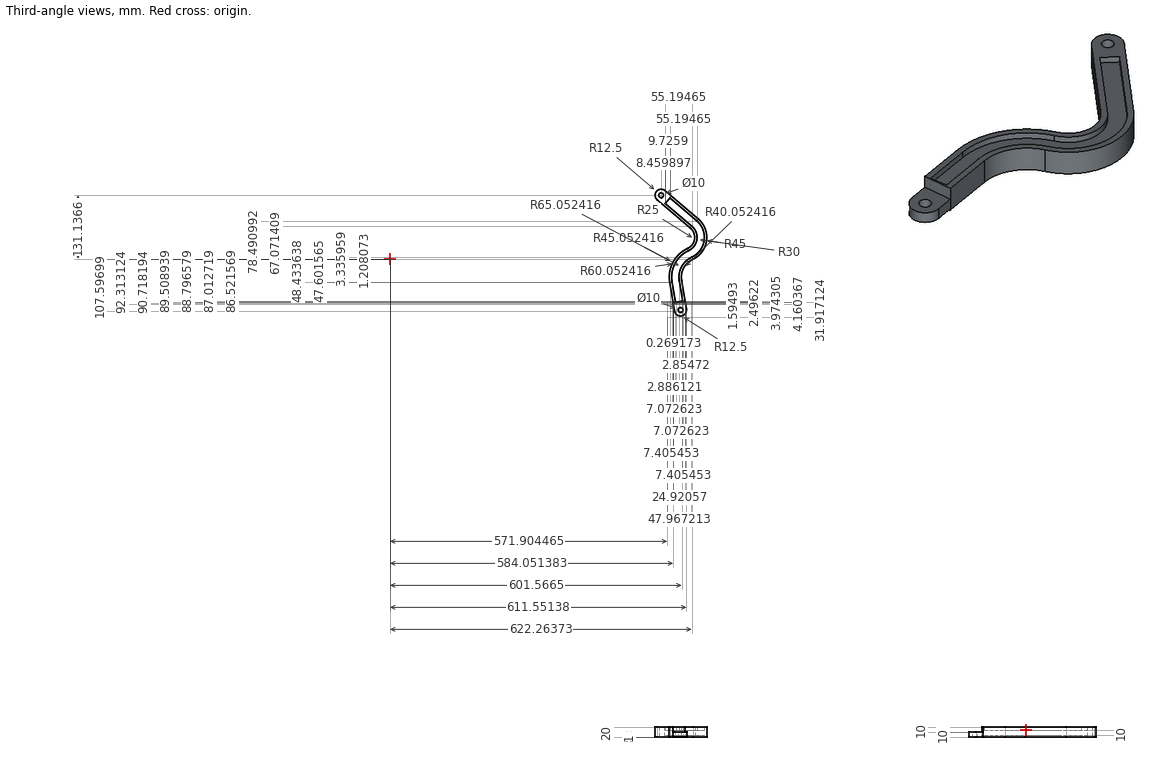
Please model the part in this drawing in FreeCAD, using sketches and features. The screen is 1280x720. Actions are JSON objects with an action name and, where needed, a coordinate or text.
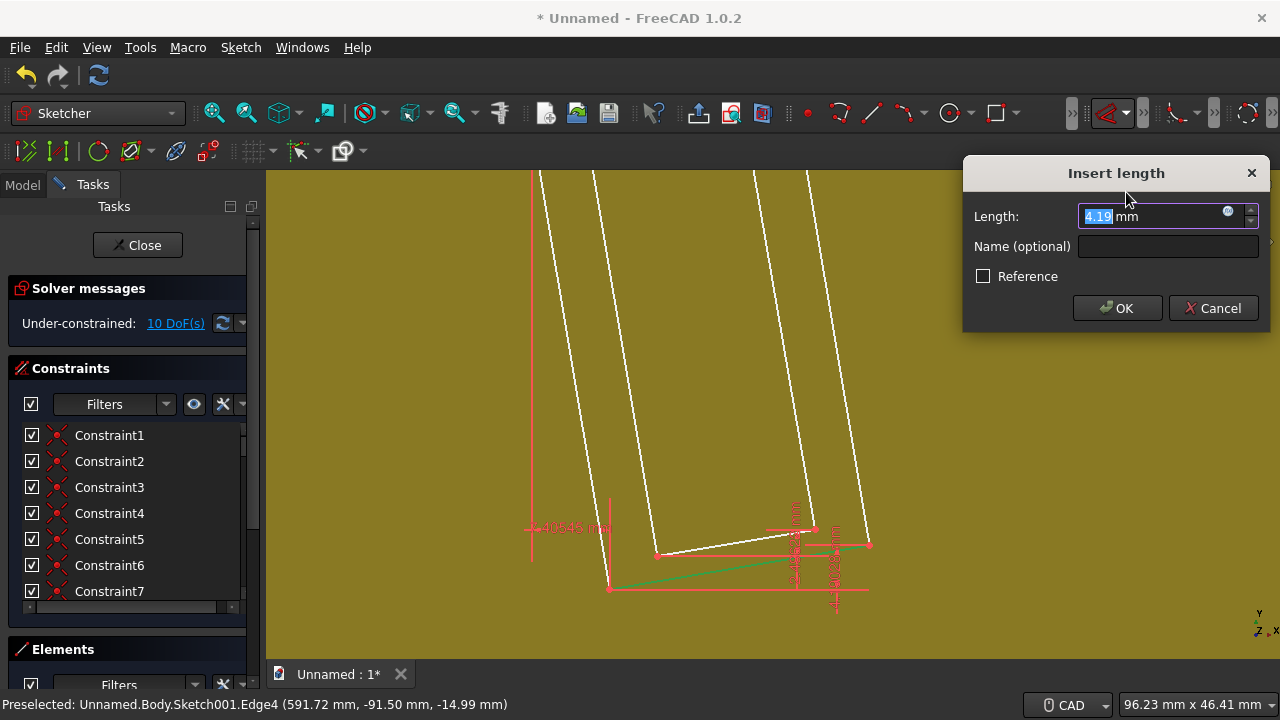
{"action": "type", "text": "4.160367"}
{"action": "key", "text": "Return"}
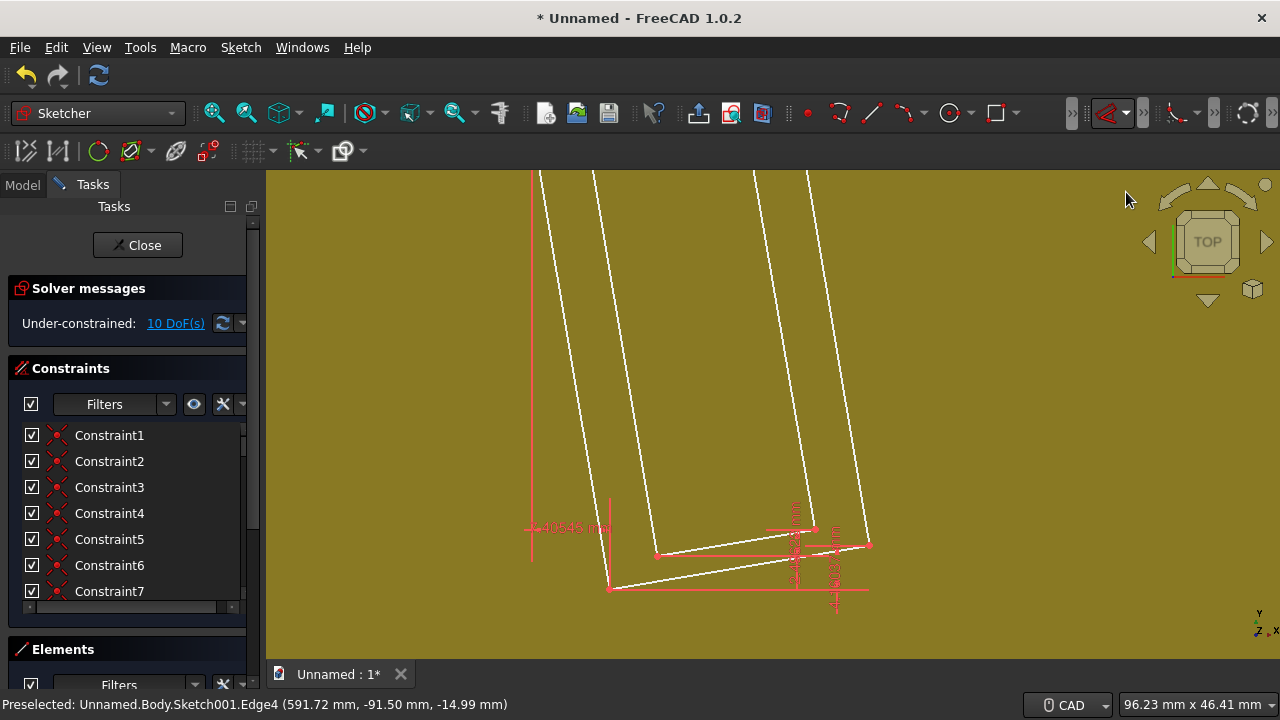
{"action": "left_click", "coordinate": [846, 406]}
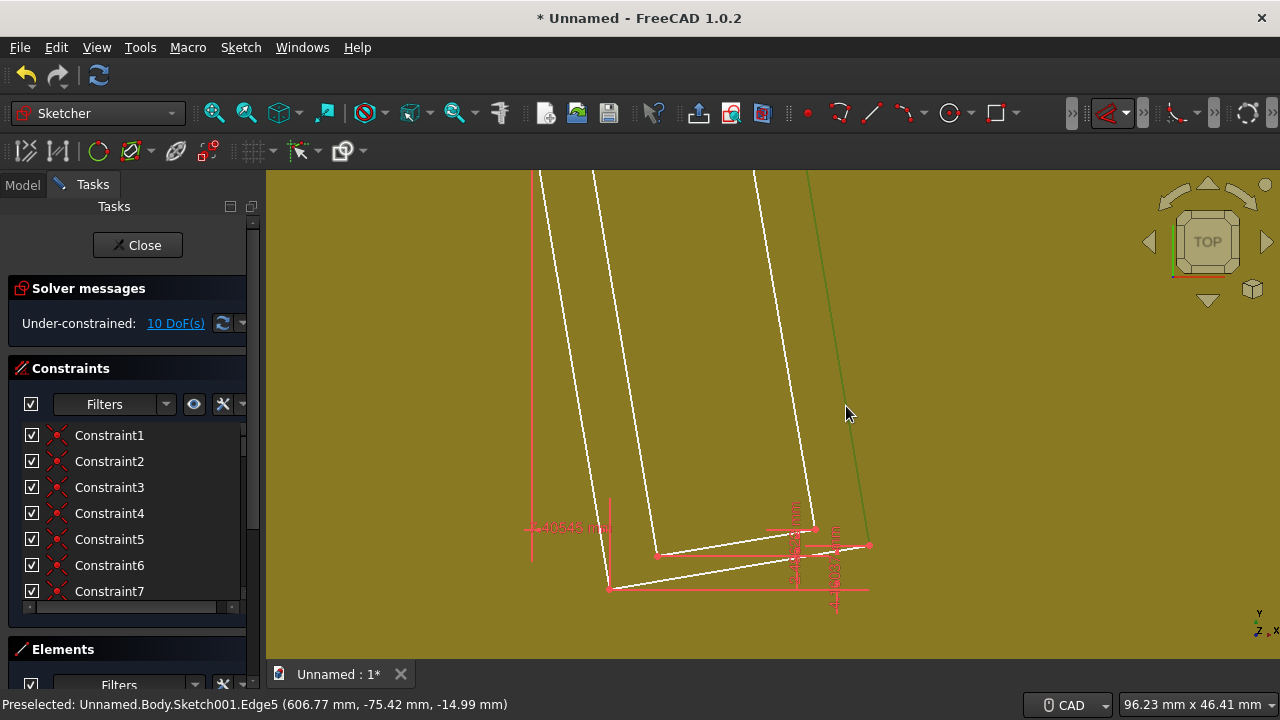
{"action": "left_click", "coordinate": [1128, 114]}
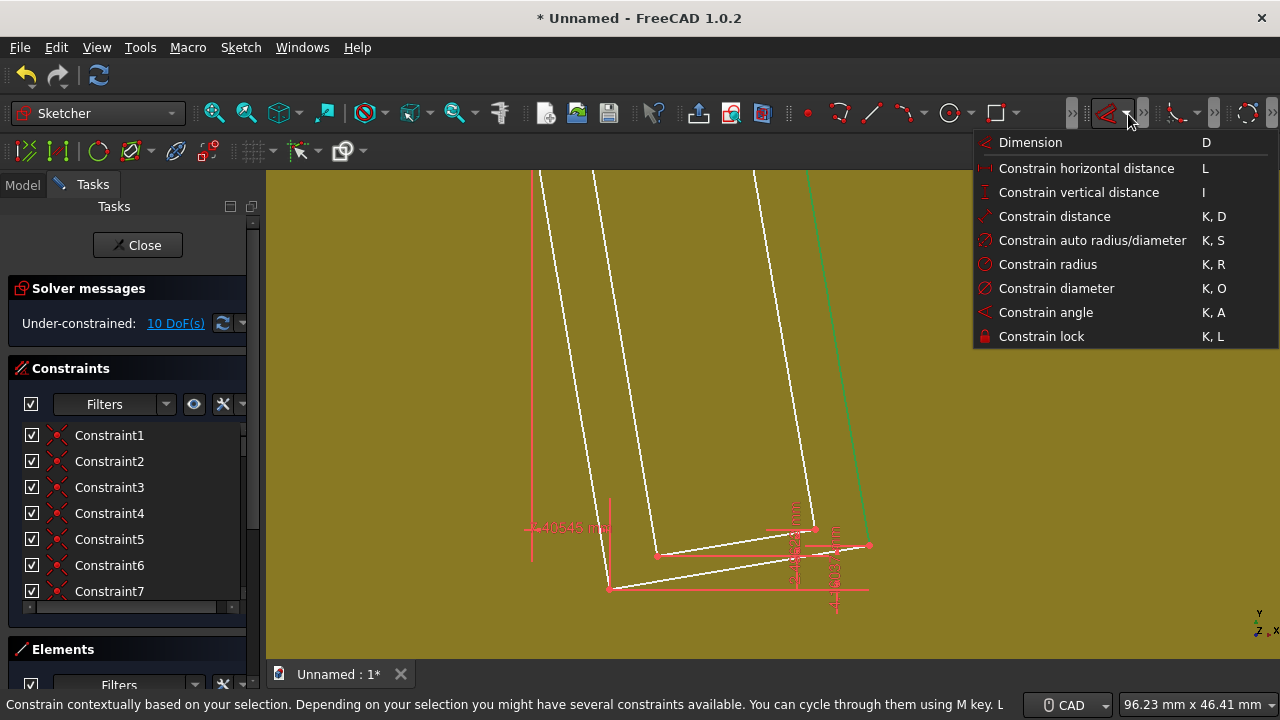
{"action": "left_click", "coordinate": [1126, 168]}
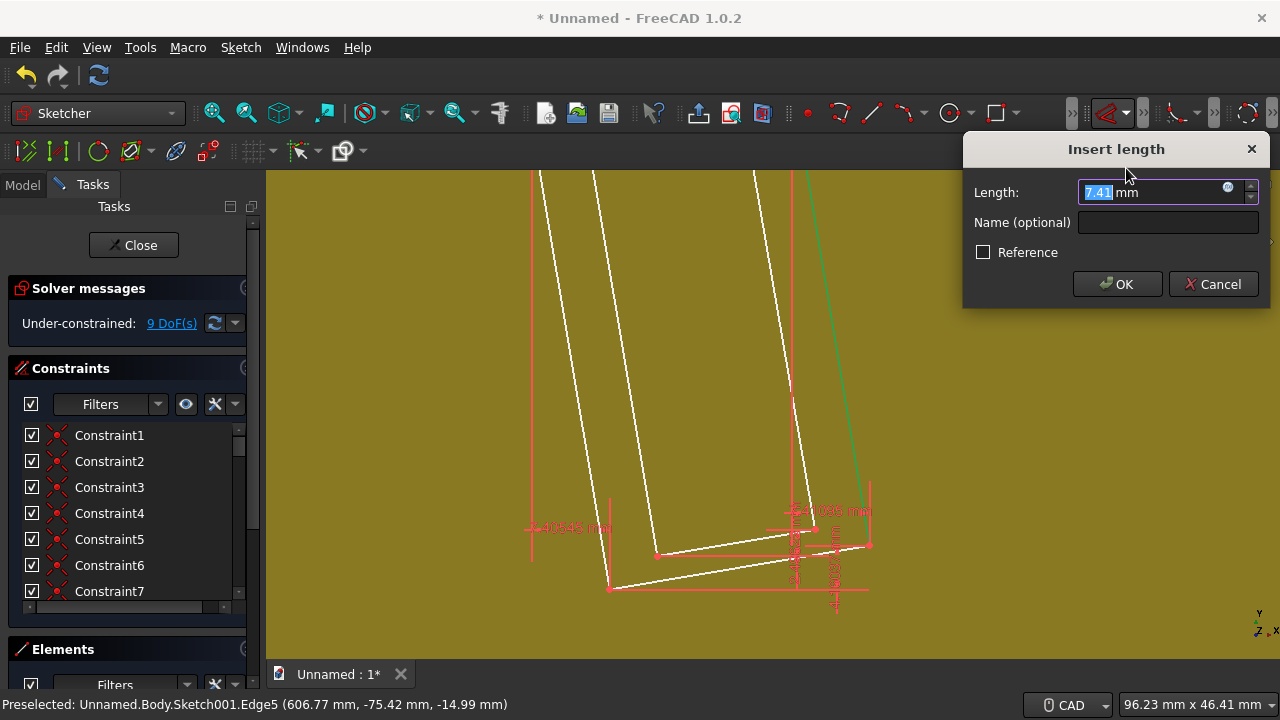
{"action": "type", "text": "7.405453"}
{"action": "key", "text": "Return"}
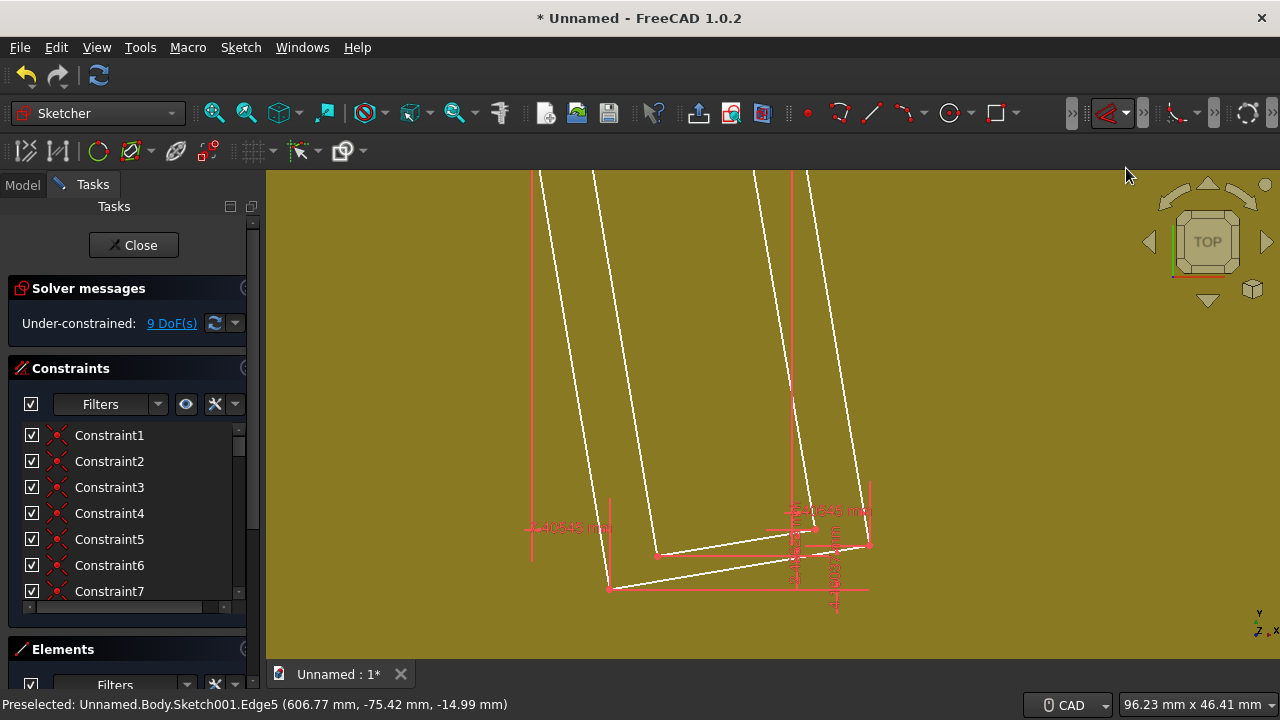
{"action": "left_click", "coordinate": [763, 223]}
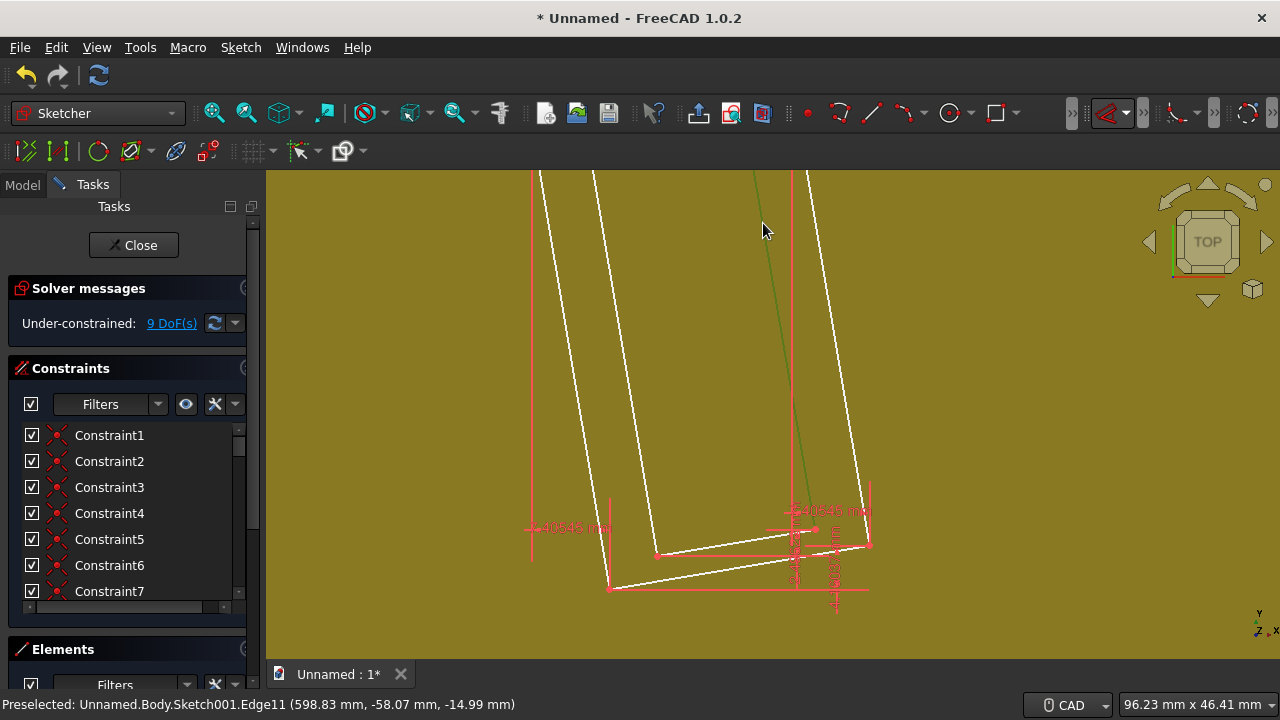
{"action": "left_click", "coordinate": [1128, 114]}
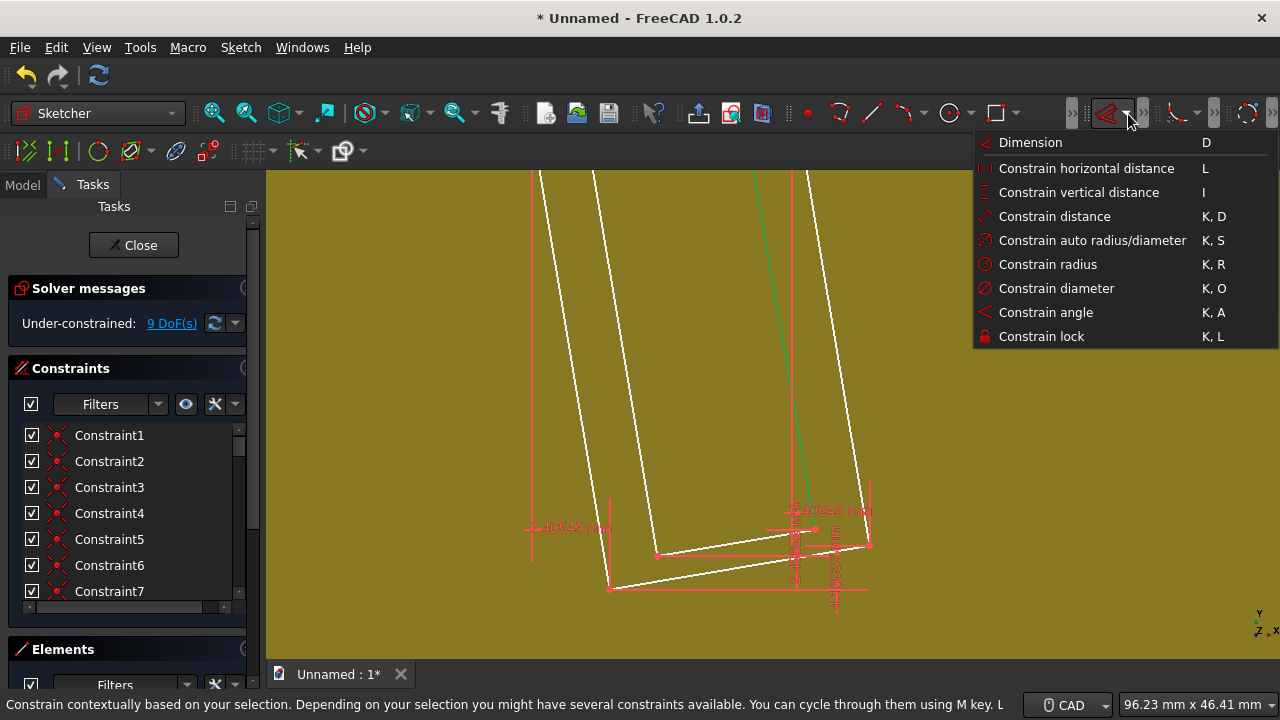
{"action": "left_click", "coordinate": [1126, 168]}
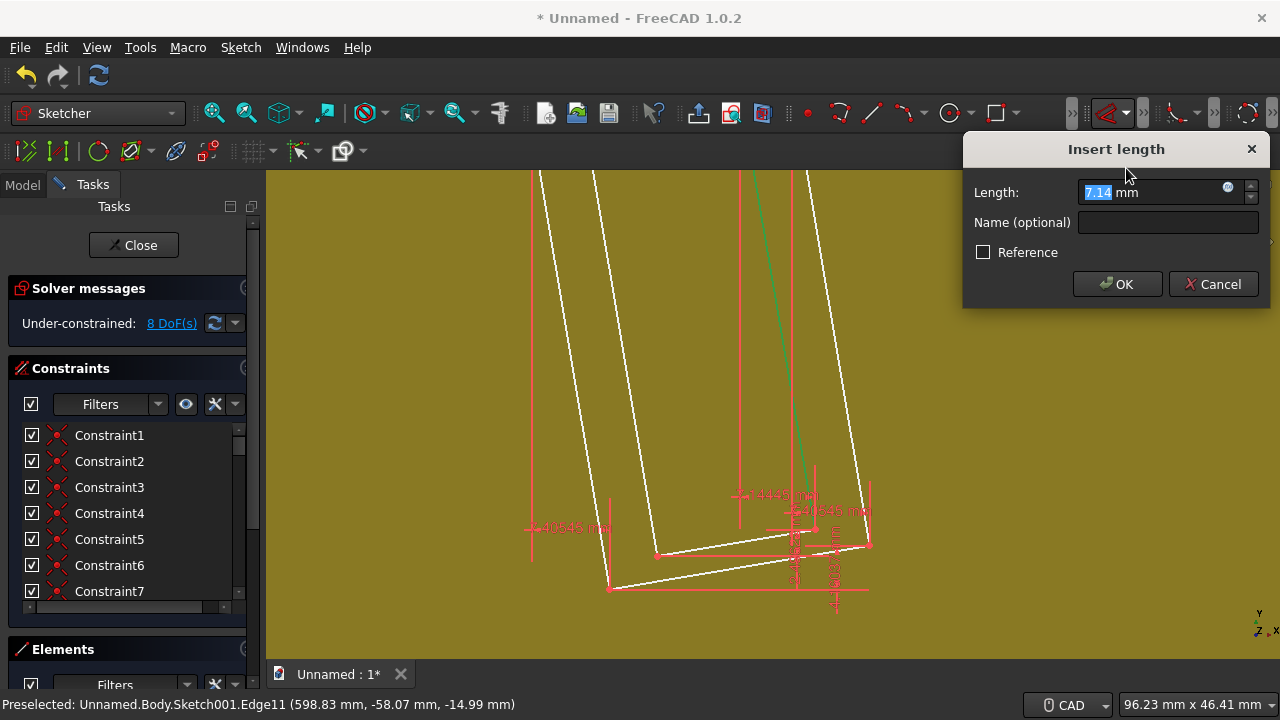
{"action": "type", "text": "7.072623"}
{"action": "key", "text": "Return"}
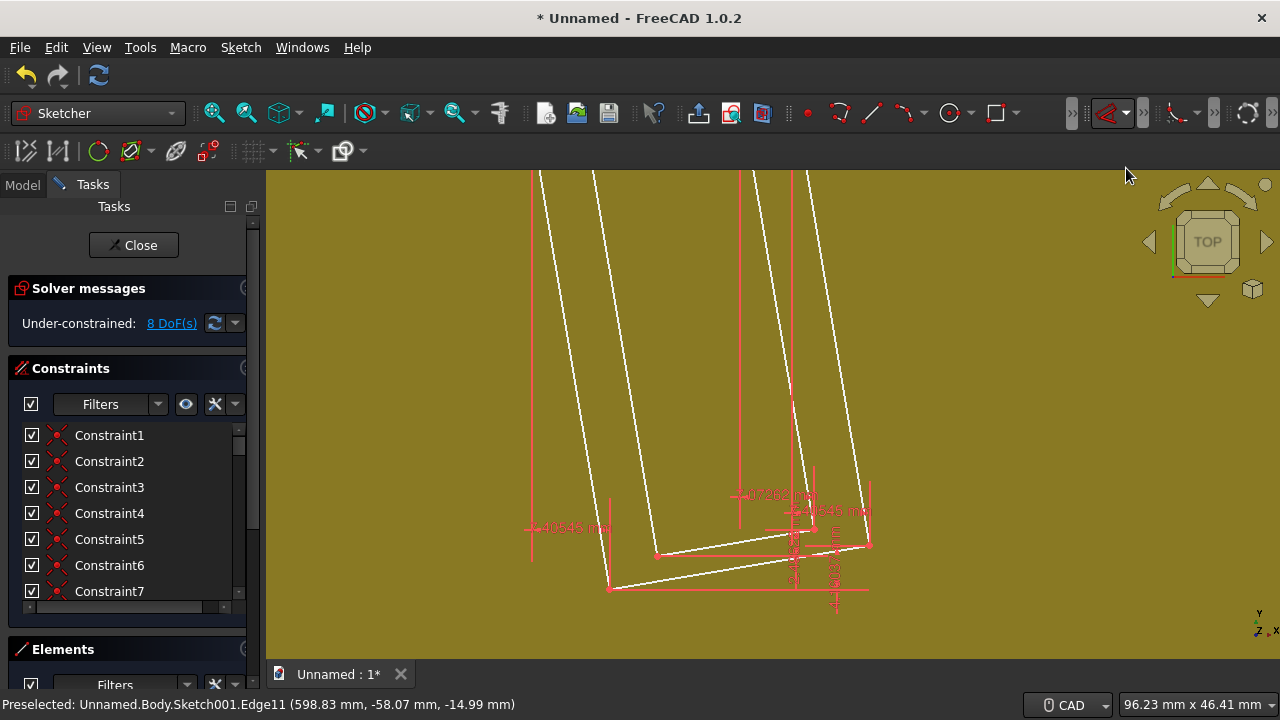
{"action": "left_click", "coordinate": [635, 424]}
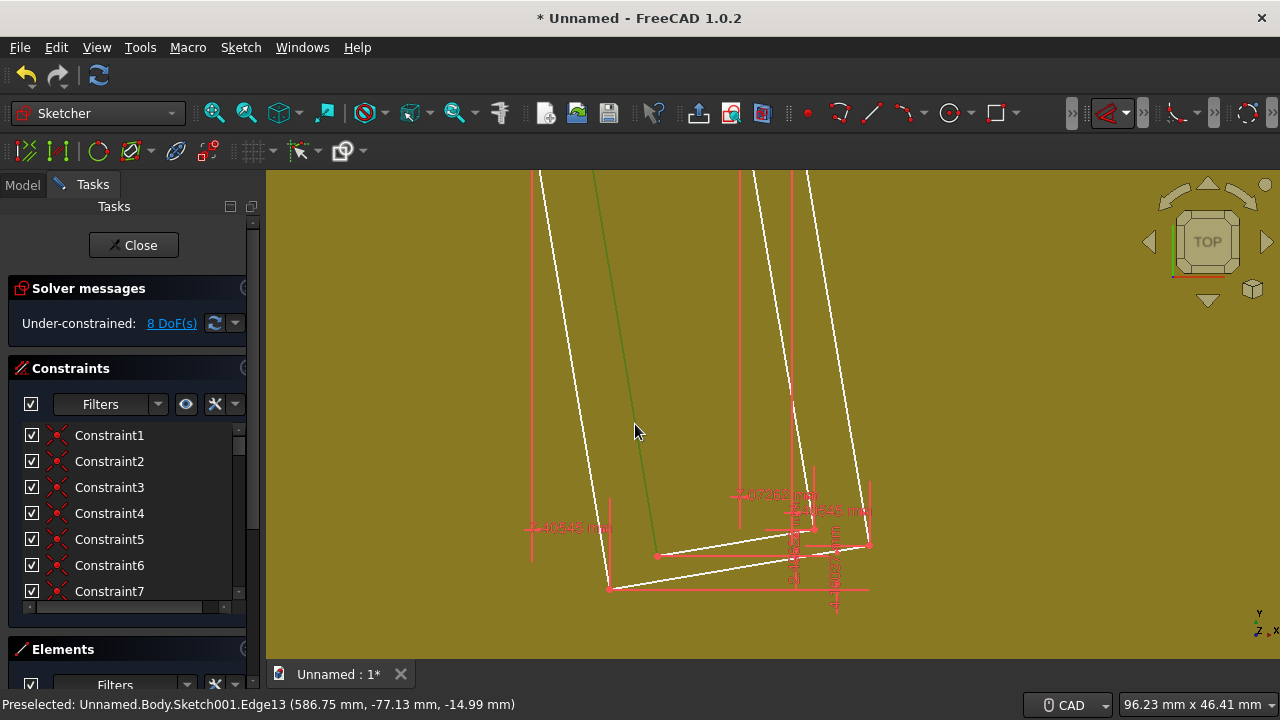
{"action": "key", "text": "l"}